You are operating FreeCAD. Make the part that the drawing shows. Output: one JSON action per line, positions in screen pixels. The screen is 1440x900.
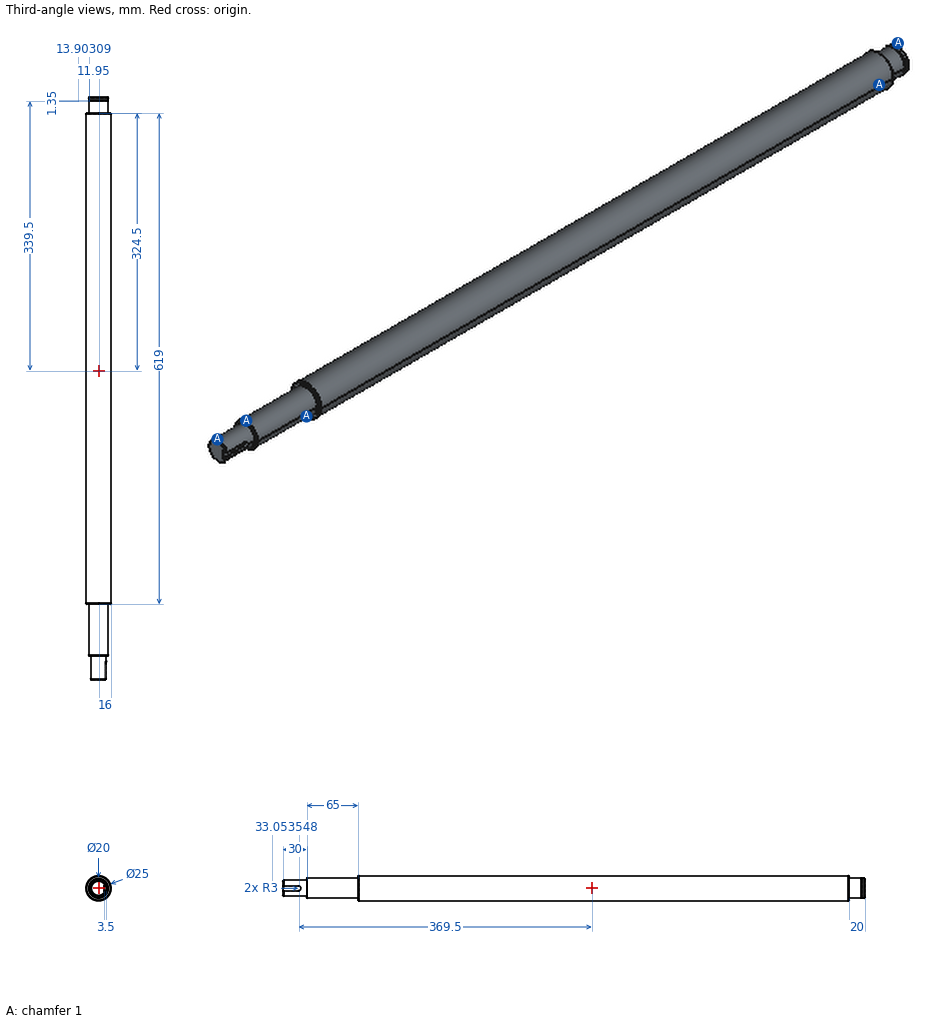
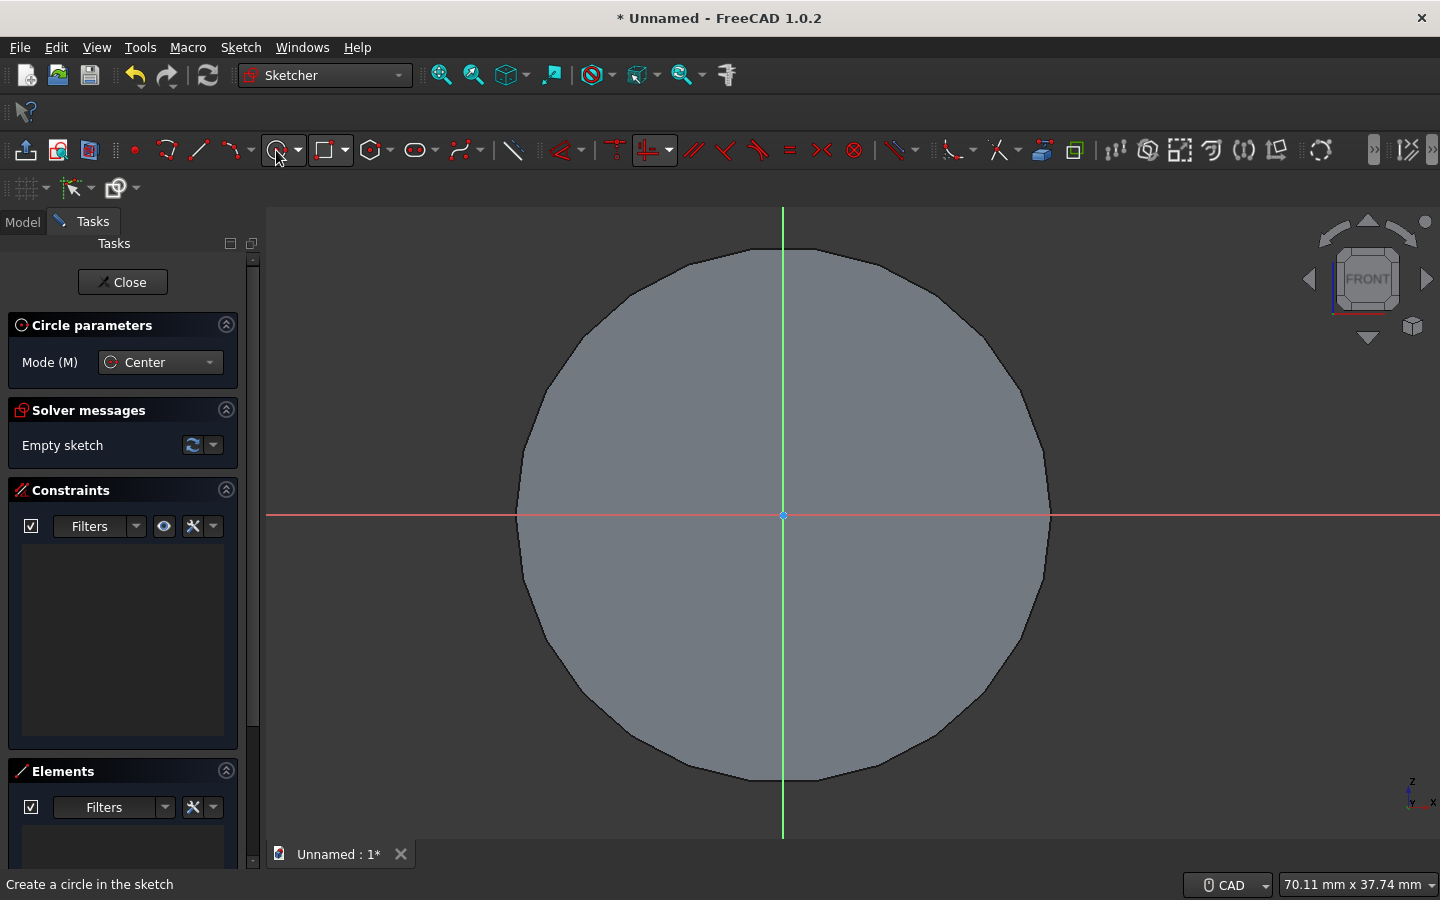
{"action": "left_click", "coordinate": [783, 515]}
{"action": "mouse_move", "coordinate": [931, 367]}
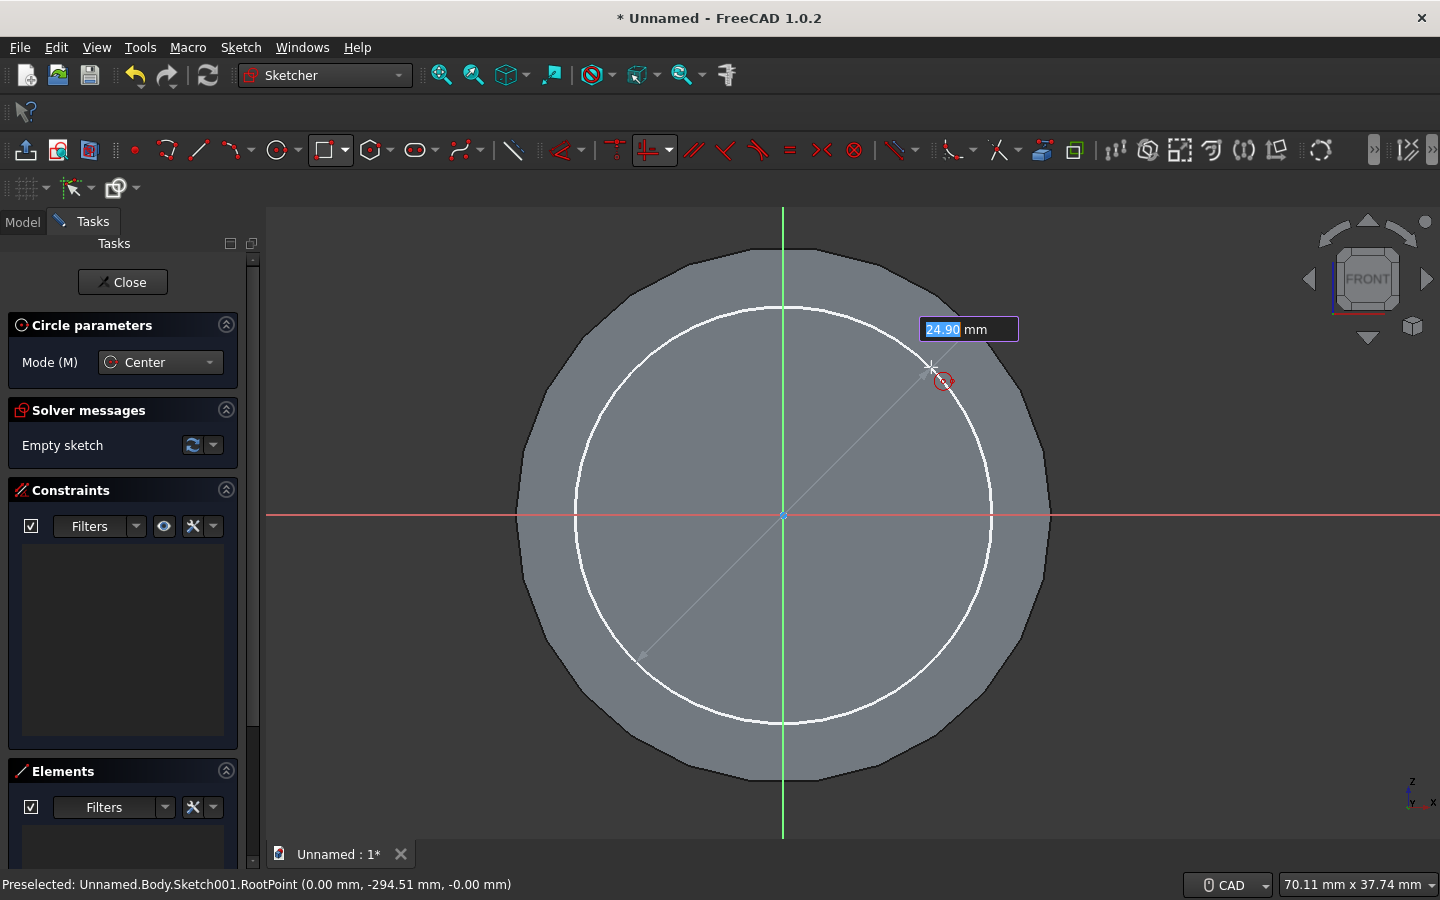
{"action": "type", "text": "25"}
{"action": "key", "text": "Return"}
{"action": "key", "text": "Escape"}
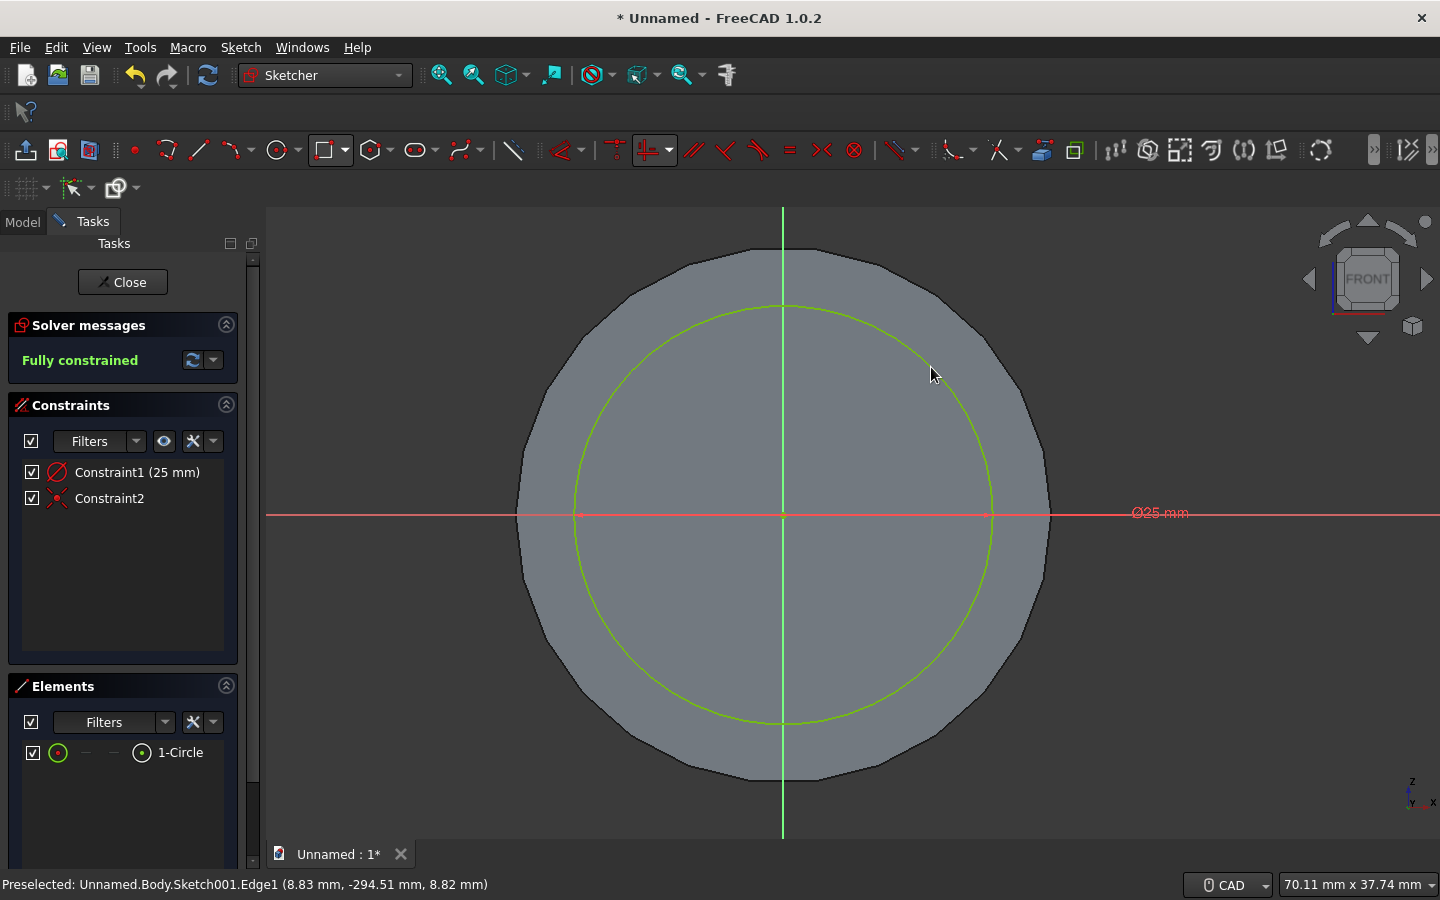
{"action": "left_click", "coordinate": [123, 282]}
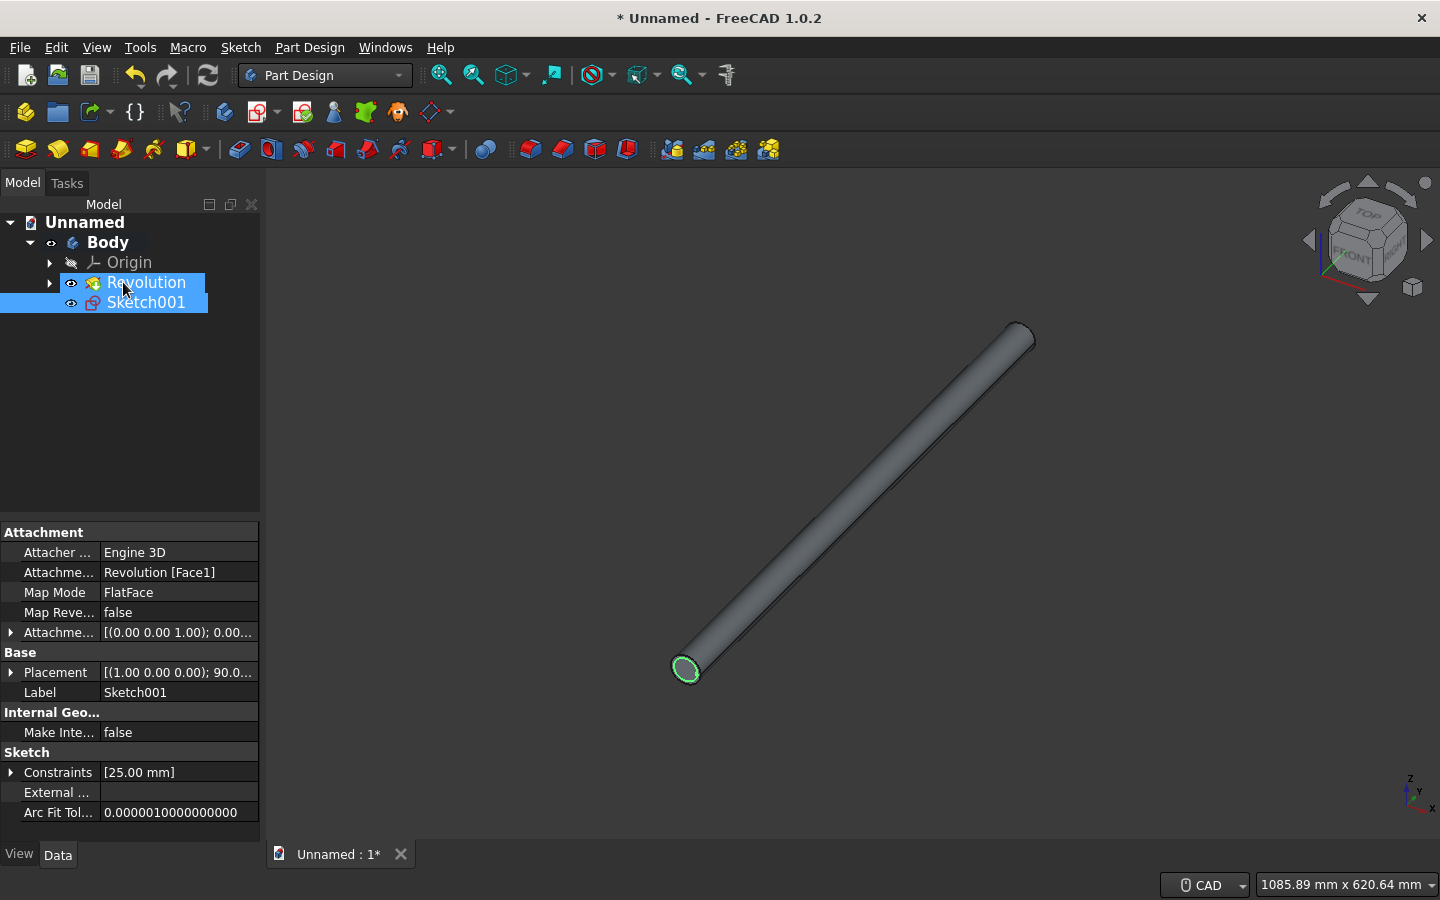
{"action": "left_click", "coordinate": [26, 150]}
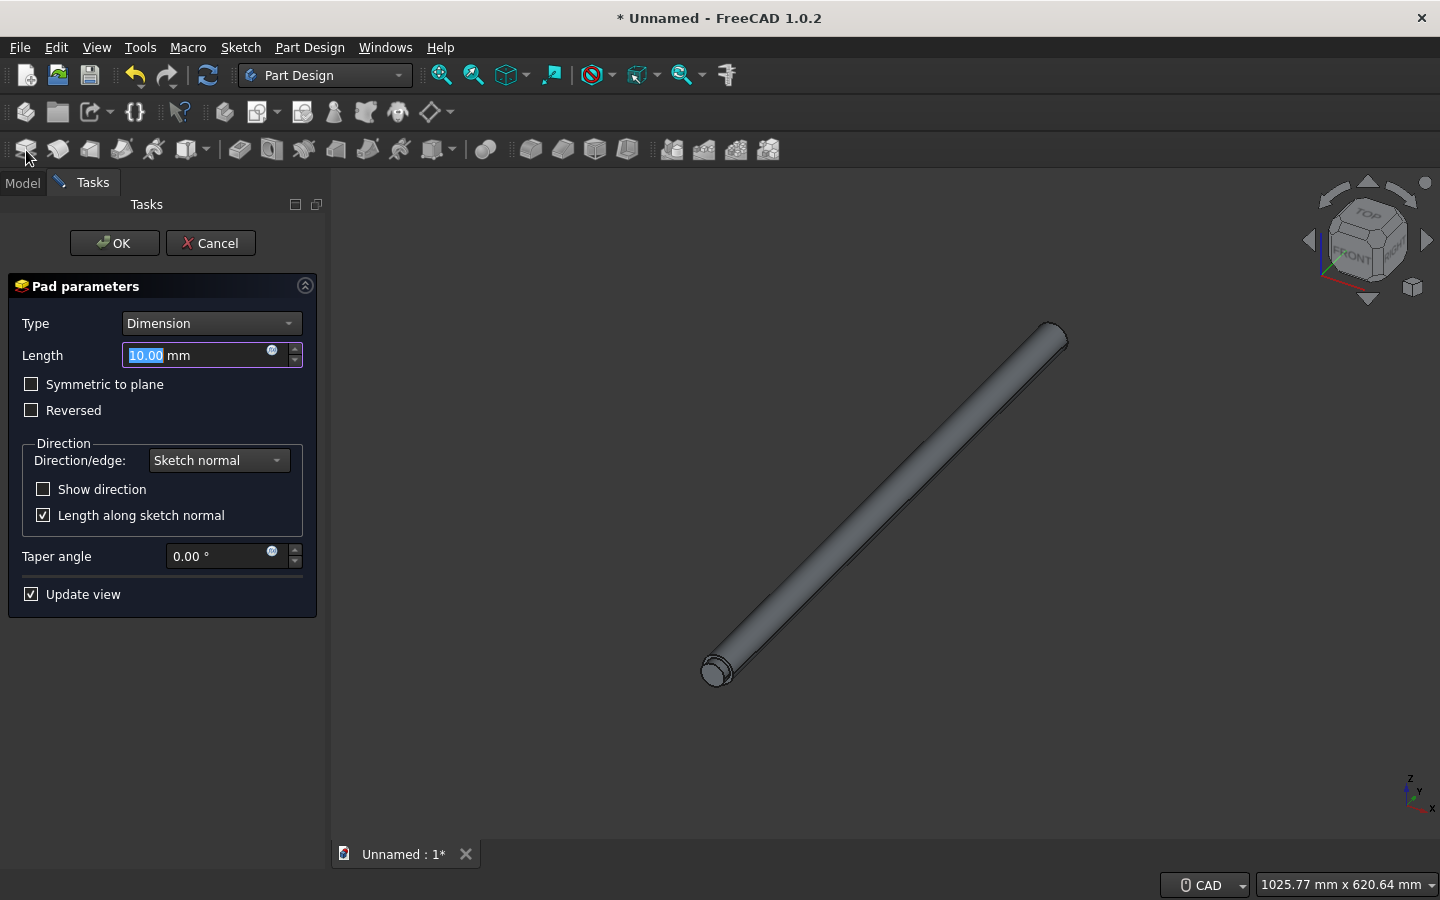
{"action": "type", "text": "65"}
{"action": "key", "text": "Tab"}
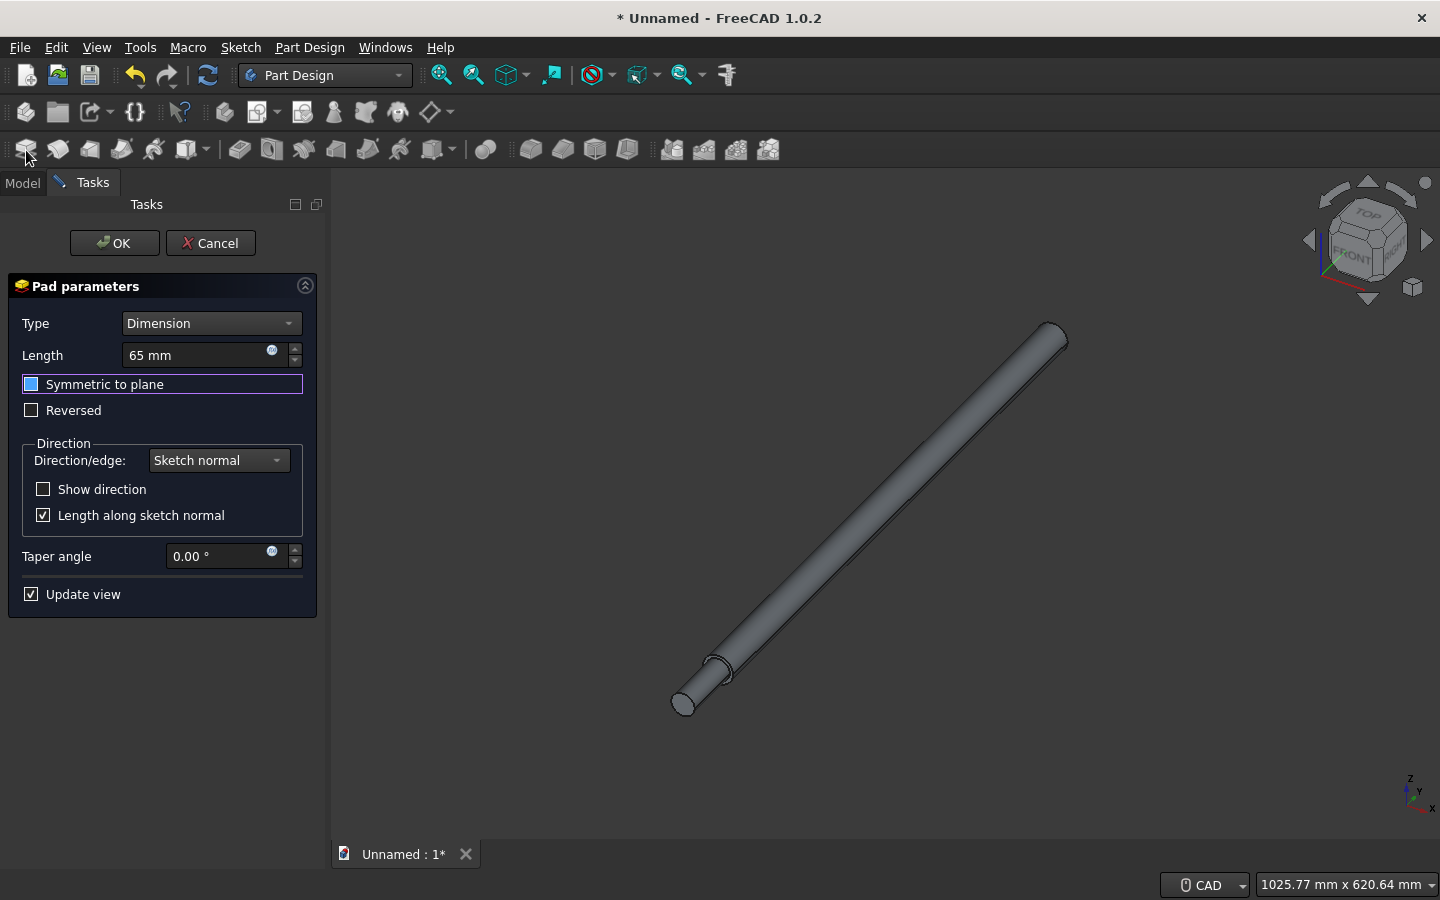
{"action": "left_click", "coordinate": [115, 243]}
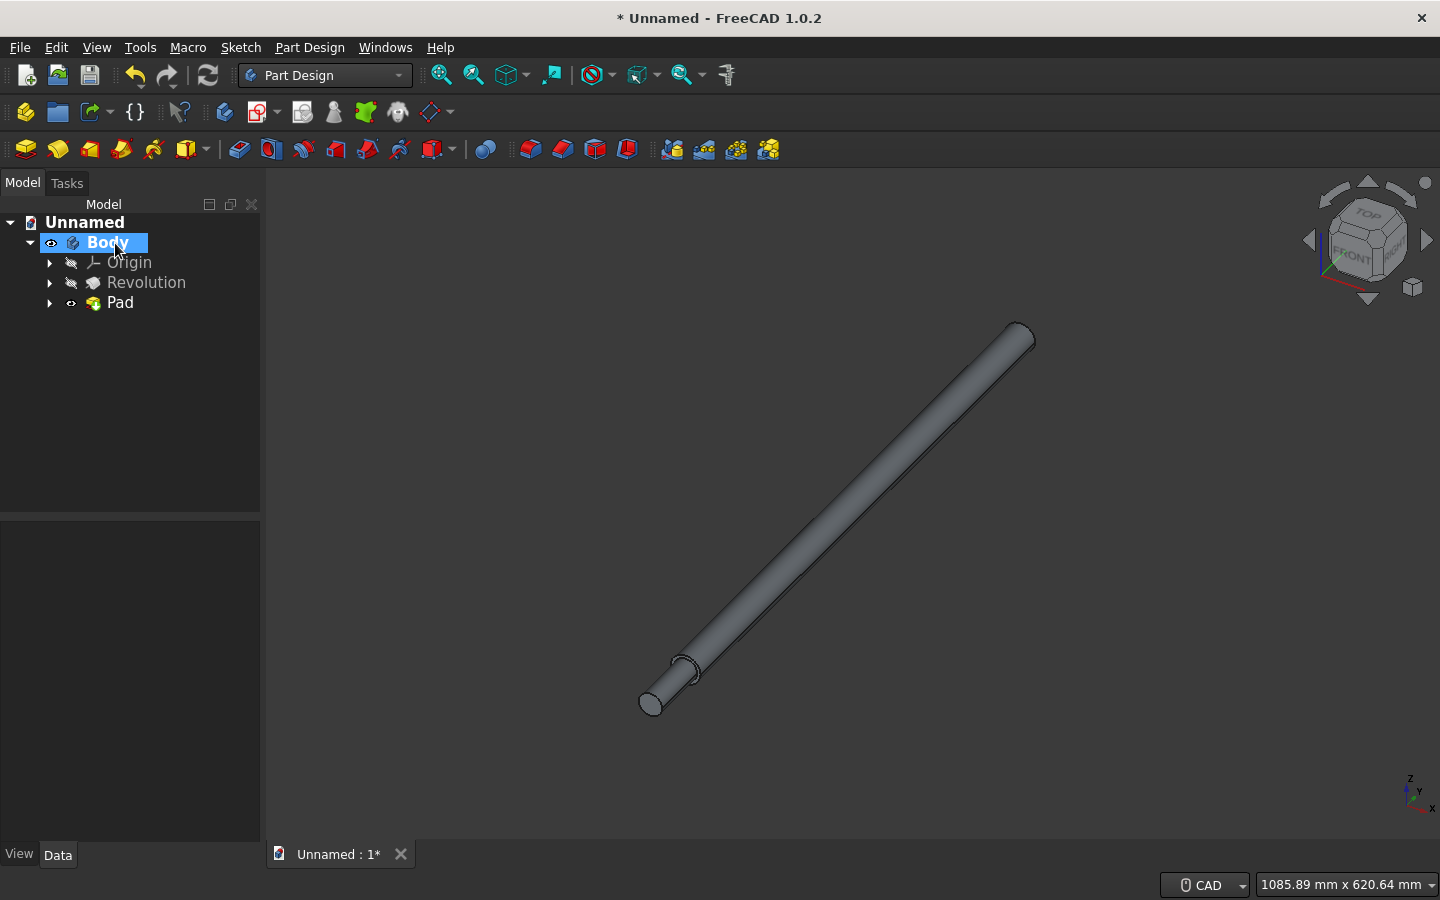
{"action": "left_click", "coordinate": [650, 704]}